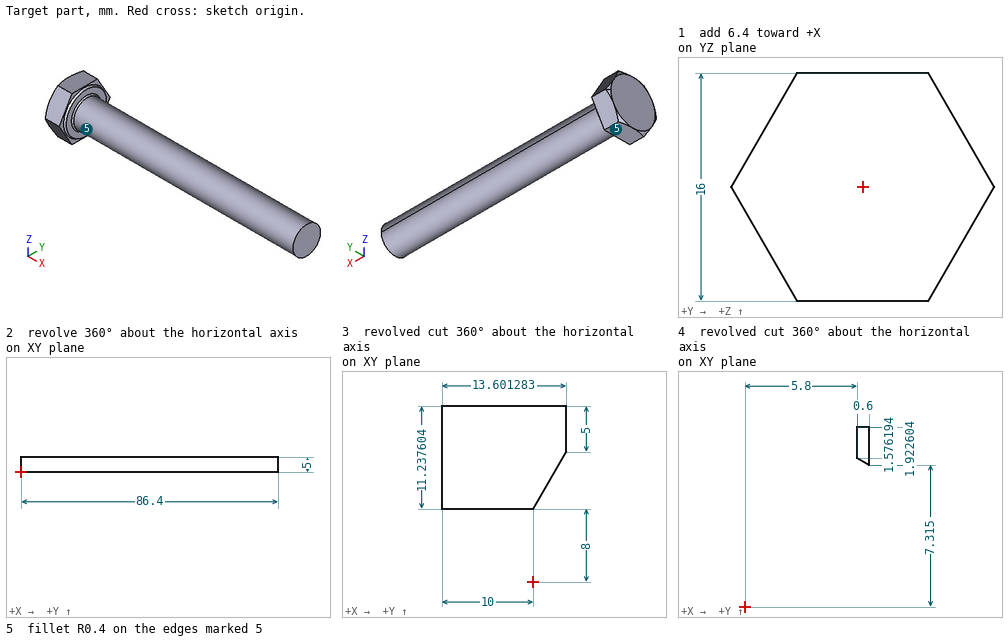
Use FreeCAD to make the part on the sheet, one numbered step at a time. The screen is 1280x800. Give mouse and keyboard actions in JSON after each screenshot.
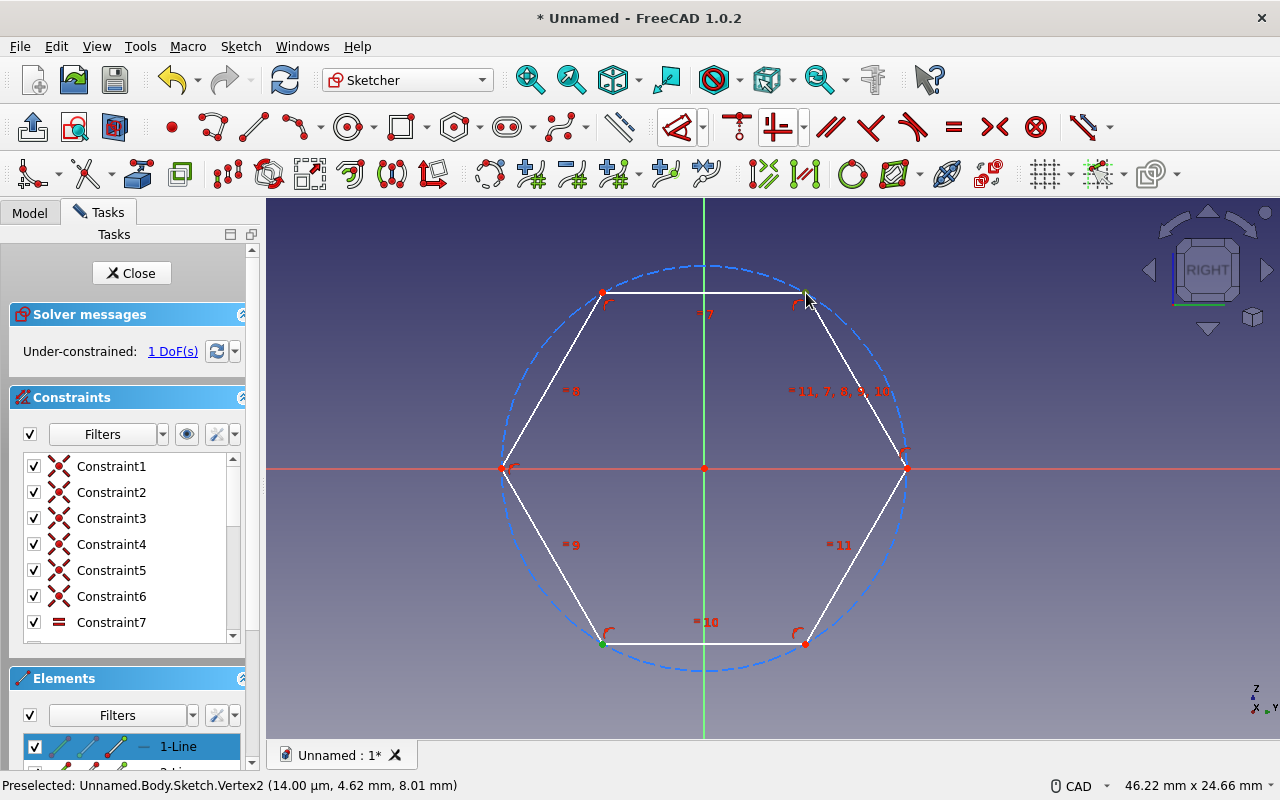
{"action": "key", "text": "i"}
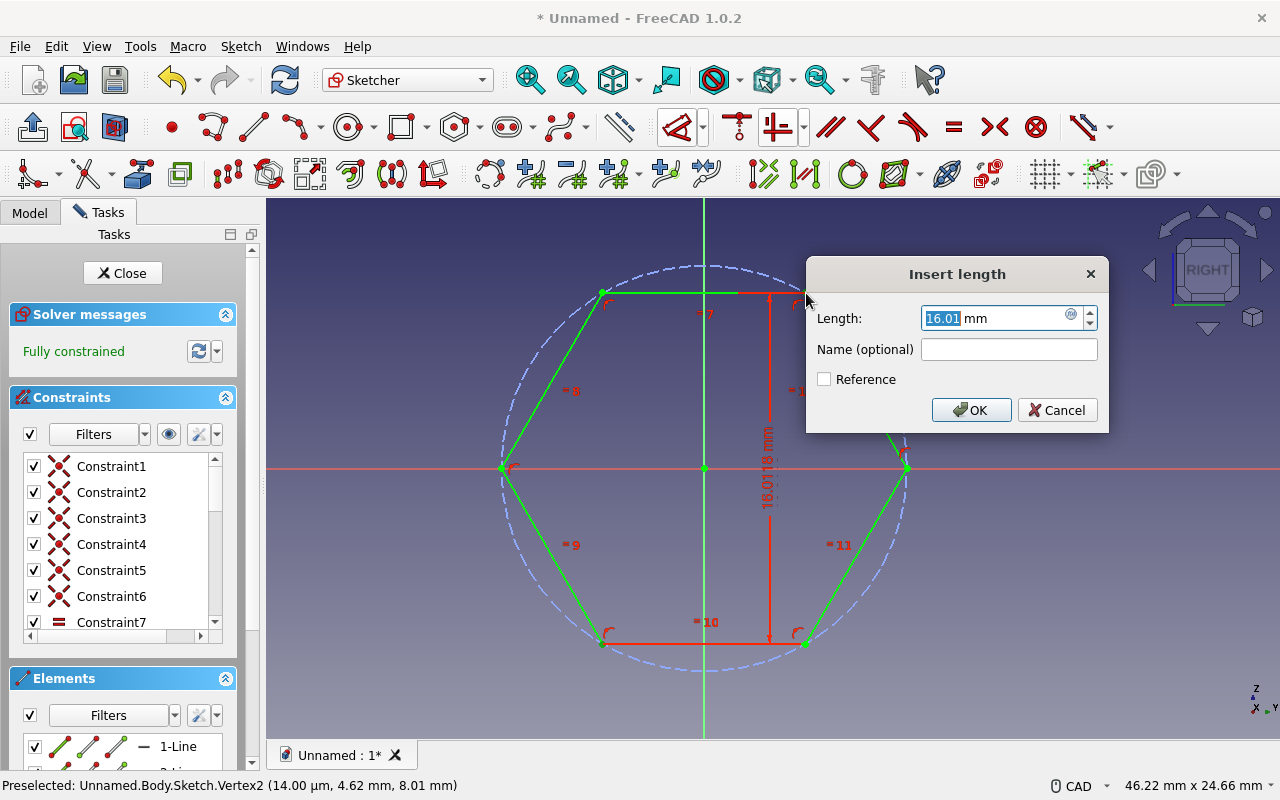
{"action": "type", "text": "16"}
{"action": "key", "text": "Return"}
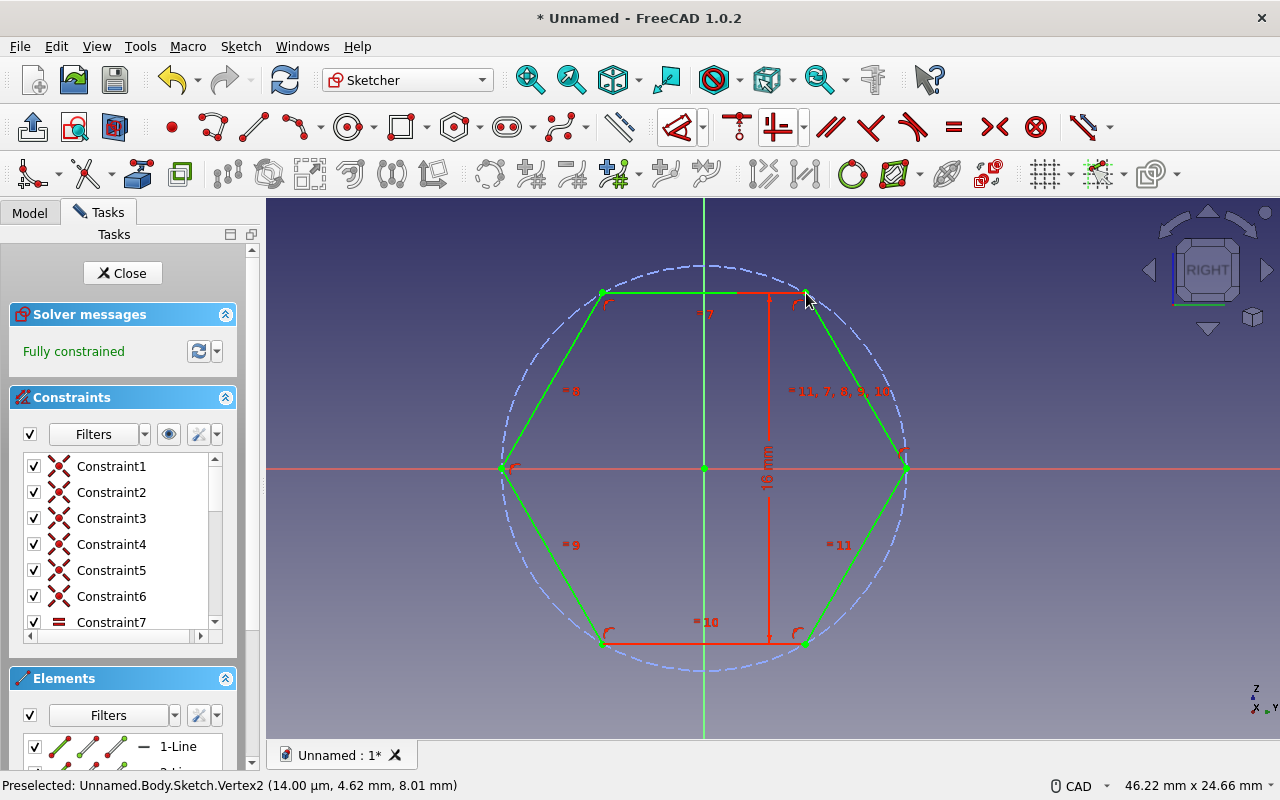
{"action": "left_click", "coordinate": [123, 273]}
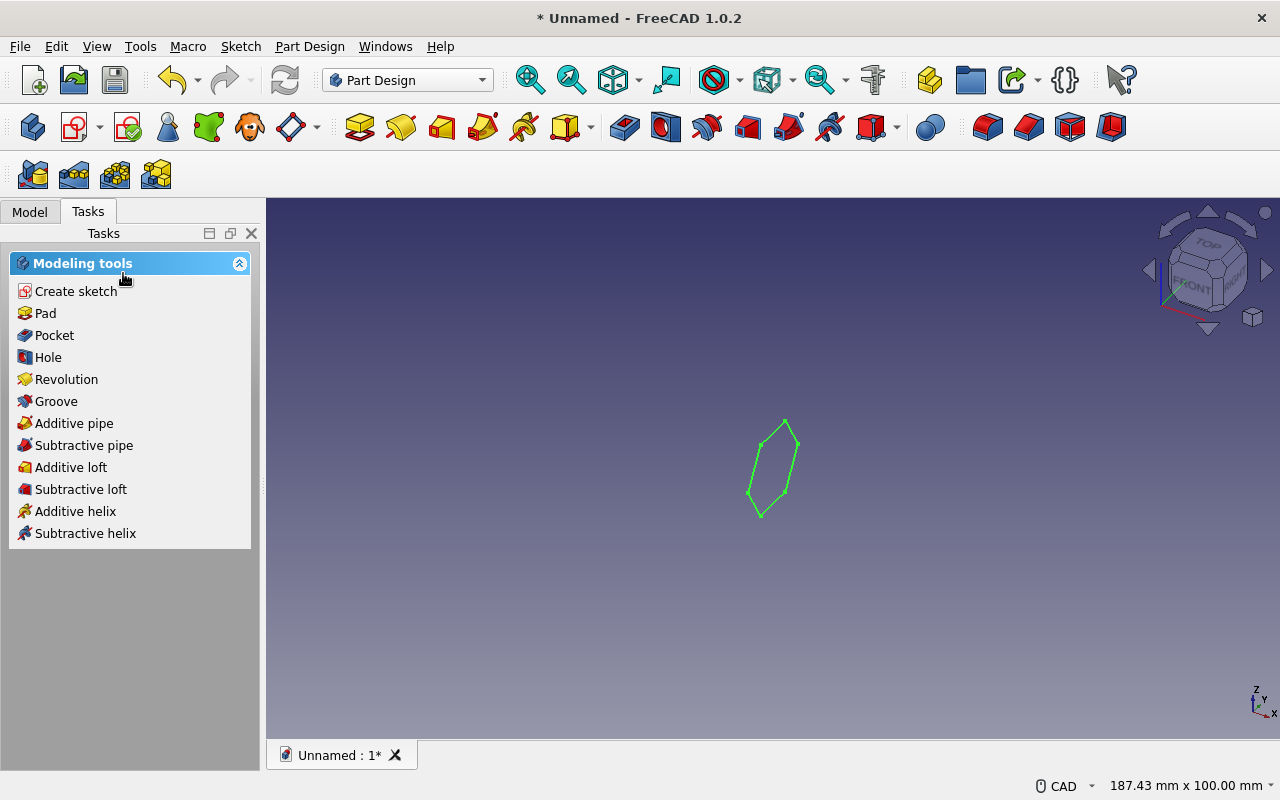
{"action": "left_click", "coordinate": [360, 128]}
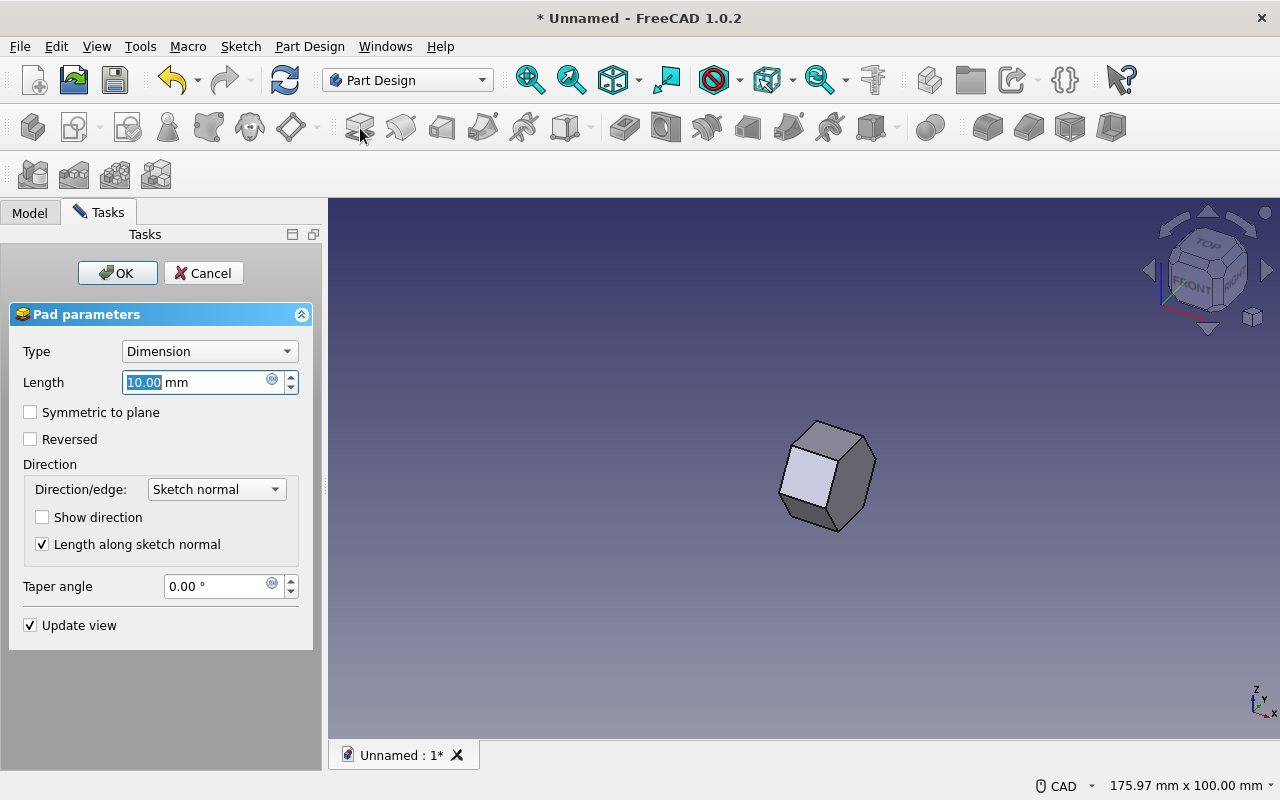
{"action": "type", "text": "6.4"}
{"action": "key", "text": "Tab"}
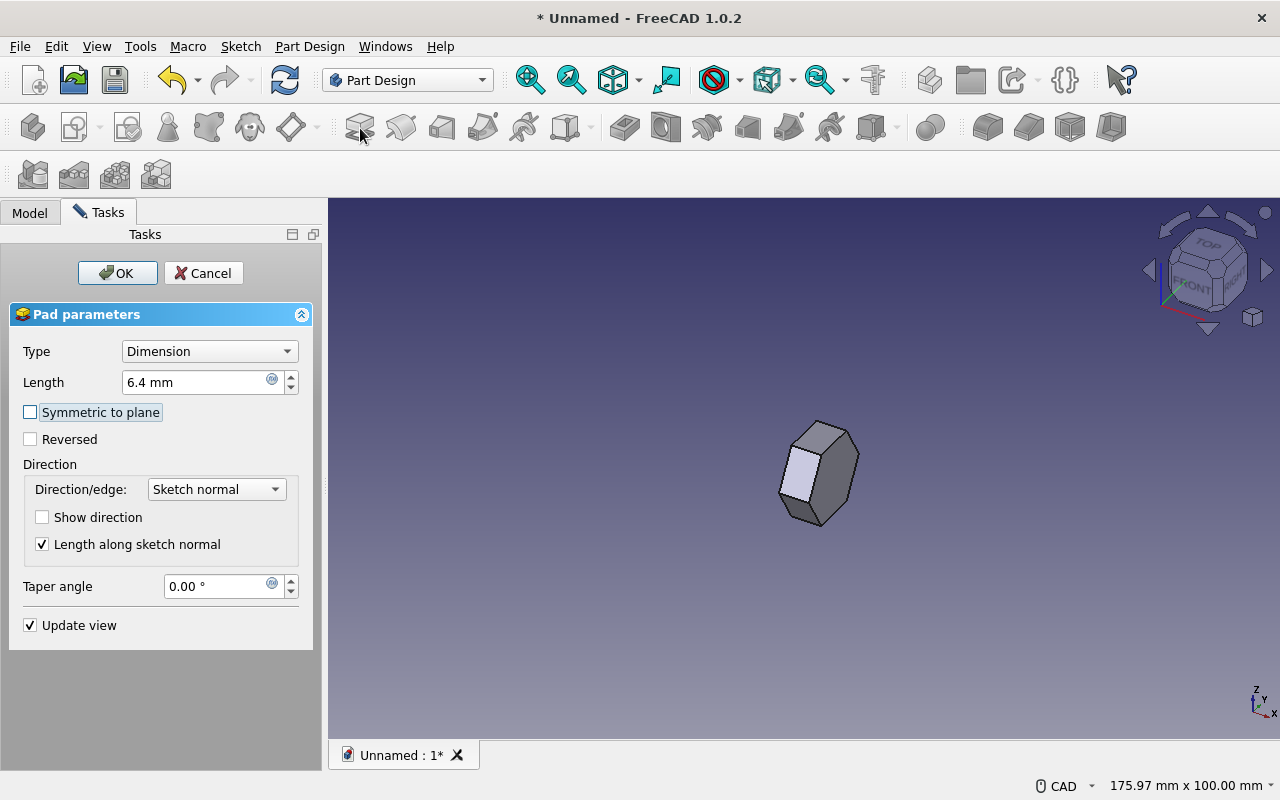
{"action": "left_click", "coordinate": [118, 273]}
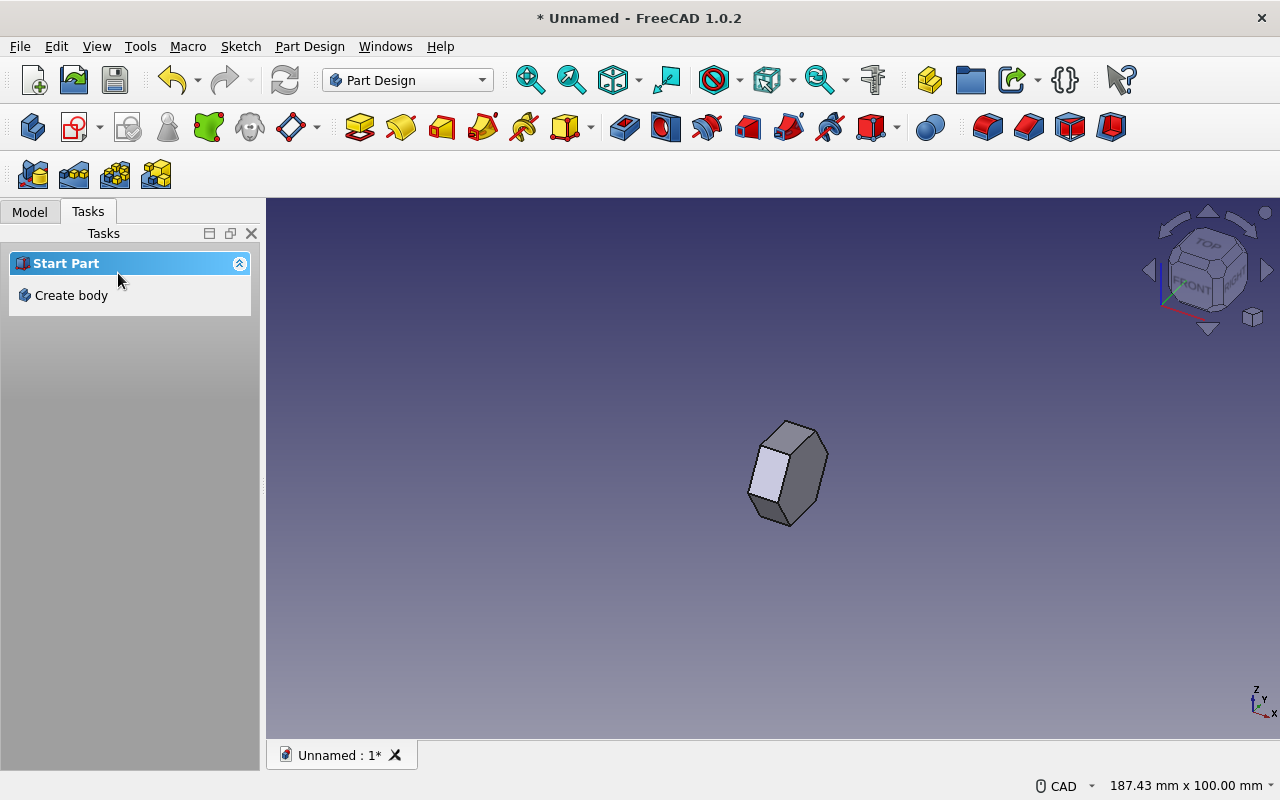
{"action": "left_click", "coordinate": [531, 80]}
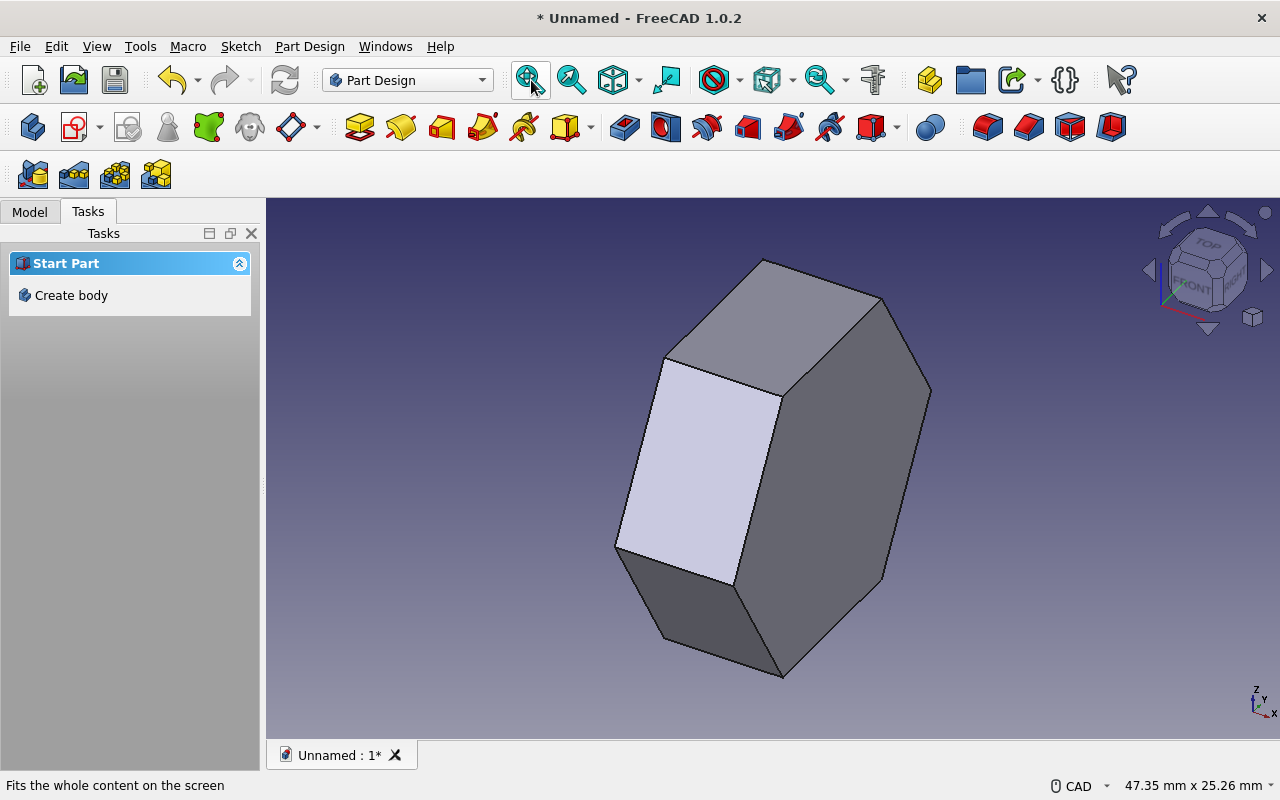
{"action": "left_click", "coordinate": [74, 128]}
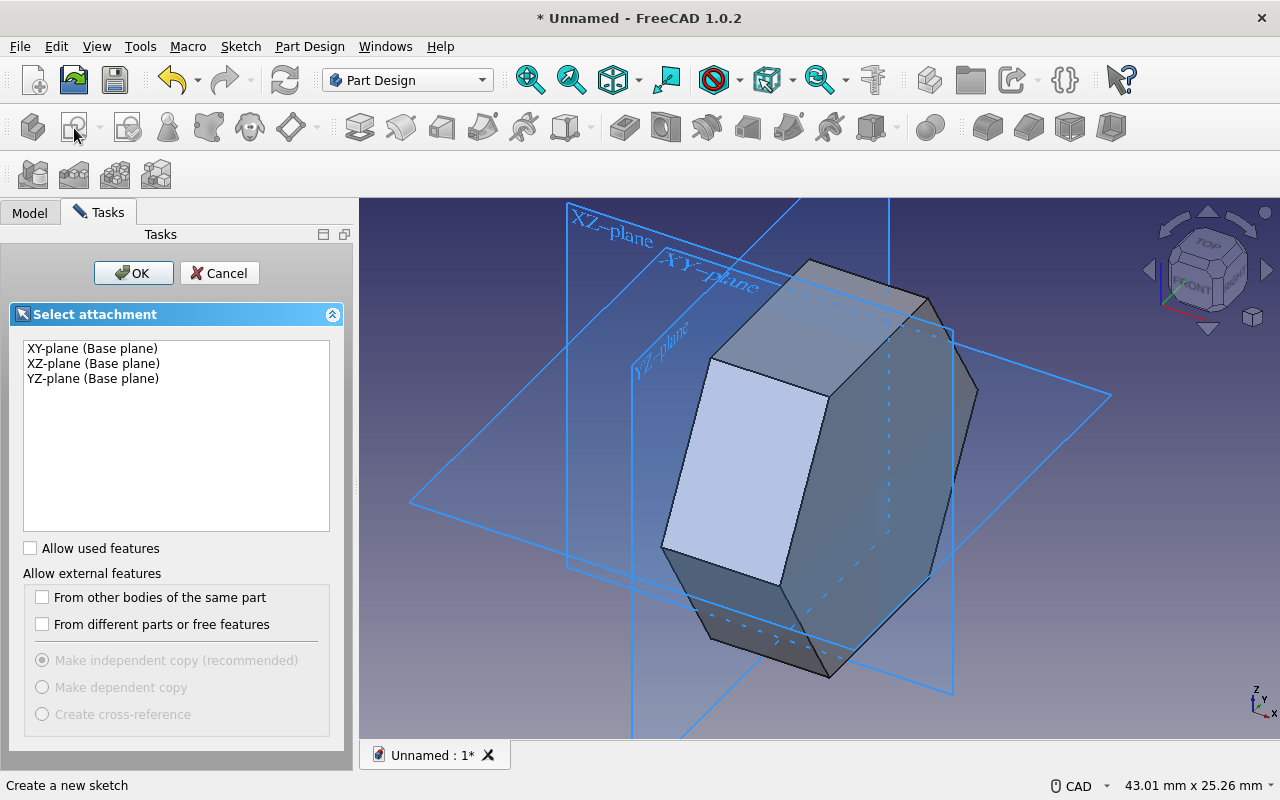
{"action": "left_click", "coordinate": [84, 348]}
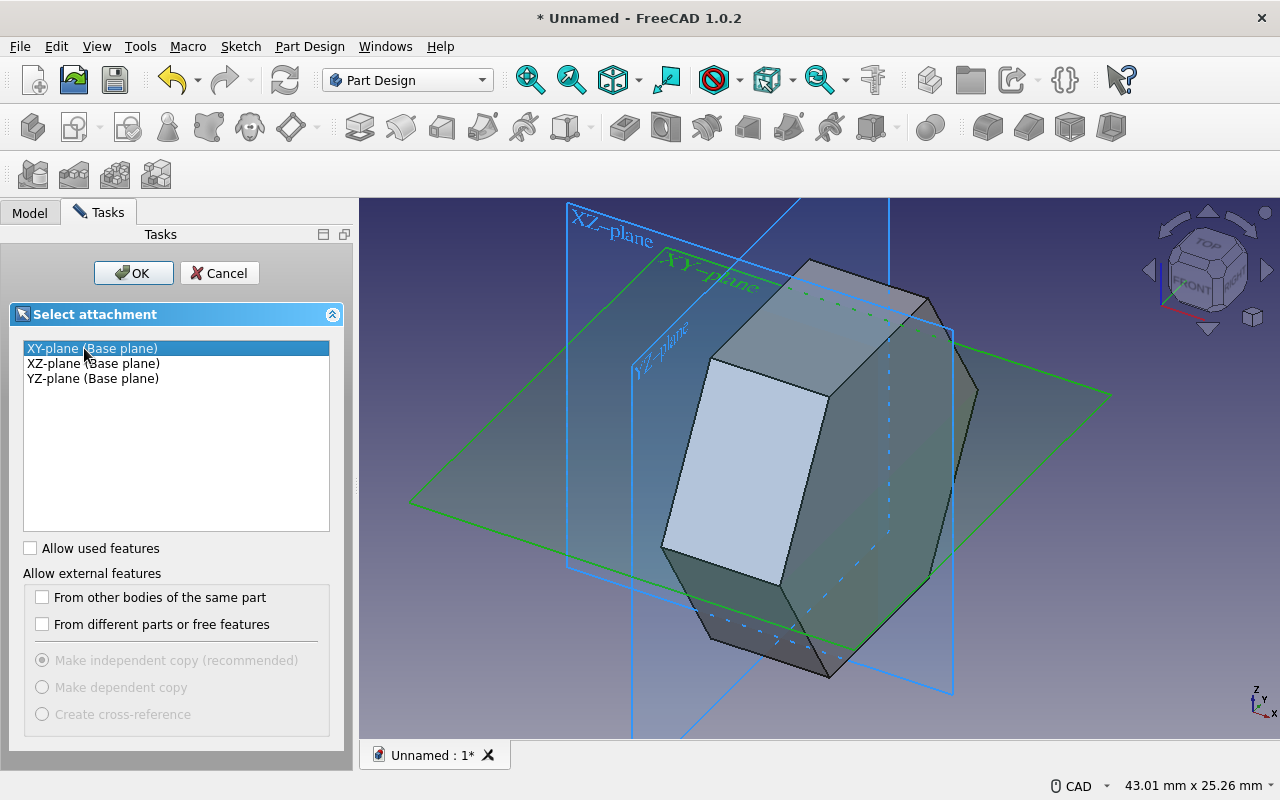
{"action": "left_click", "coordinate": [134, 273]}